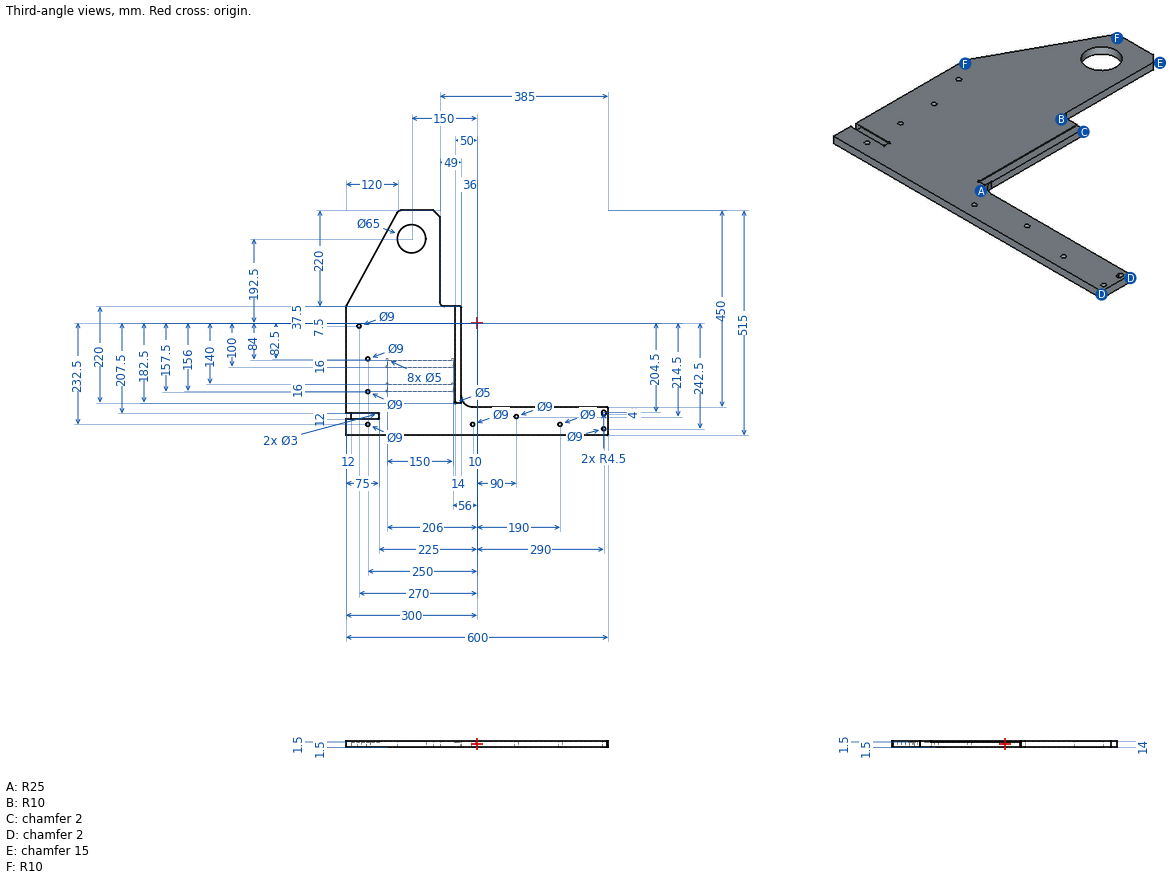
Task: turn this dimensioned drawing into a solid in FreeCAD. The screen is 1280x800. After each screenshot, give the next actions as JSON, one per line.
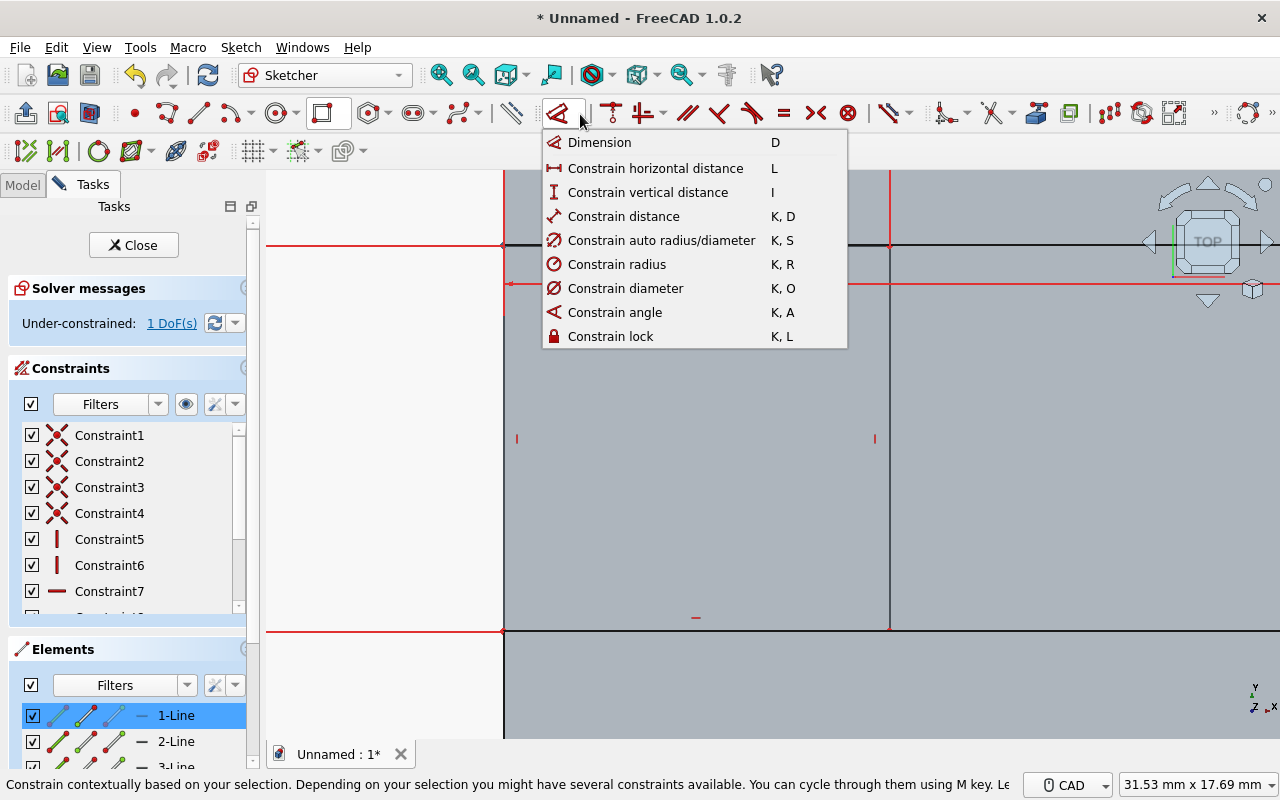
{"action": "left_click", "coordinate": [695, 192]}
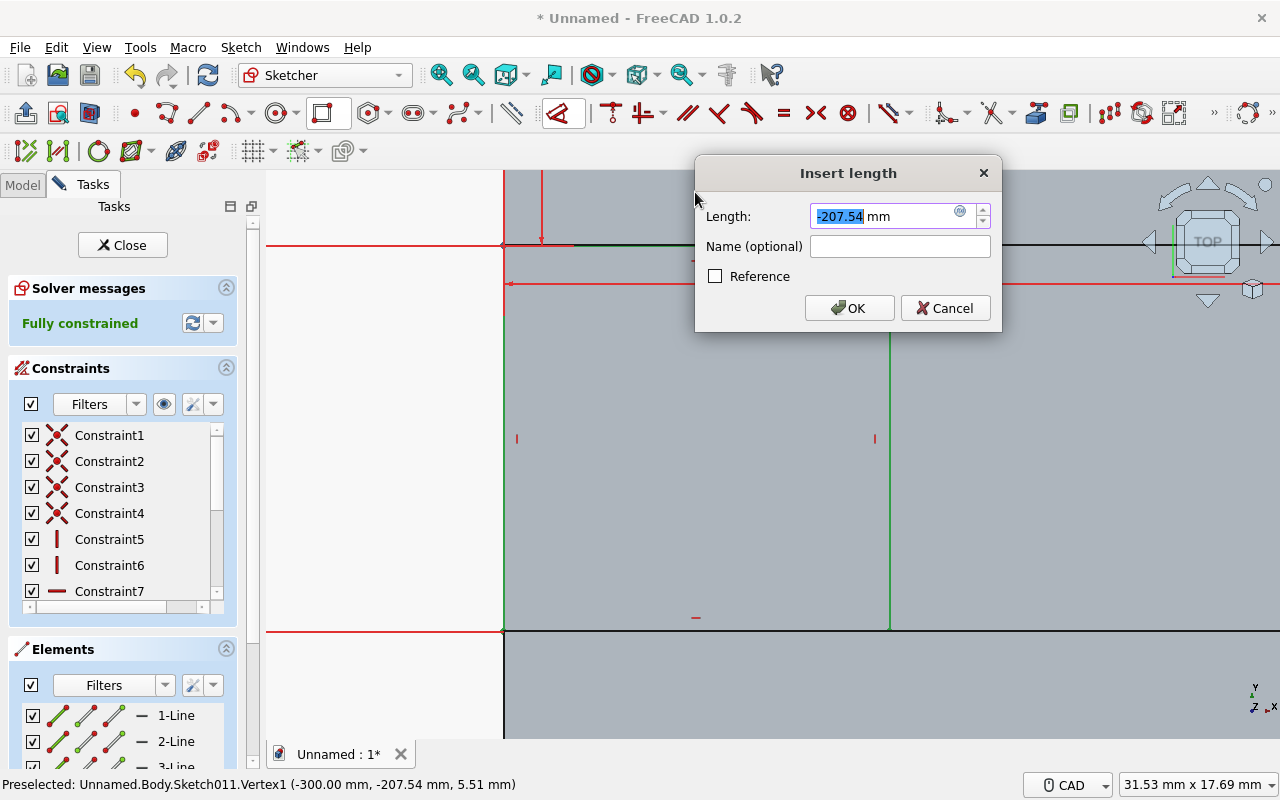
{"action": "type", "text": "-207.5"}
{"action": "key", "text": "Return"}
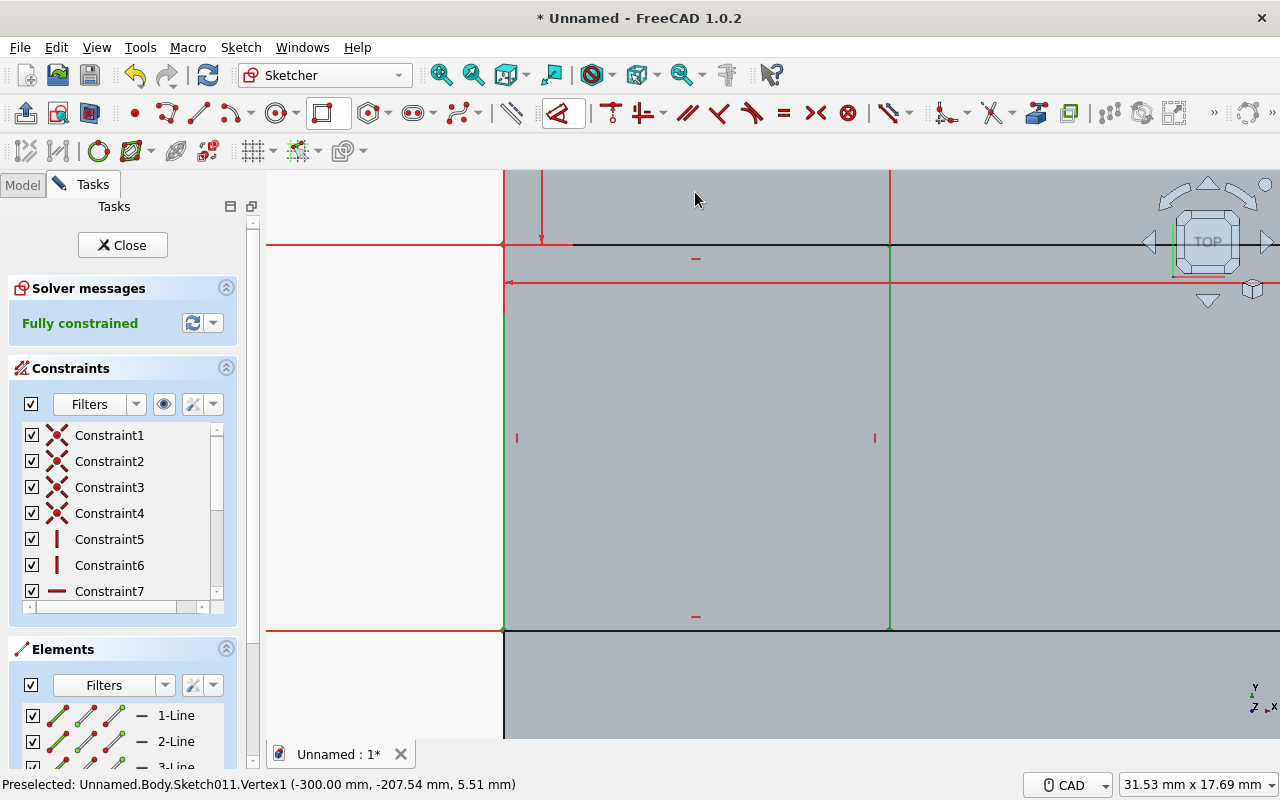
{"action": "left_click", "coordinate": [123, 245]}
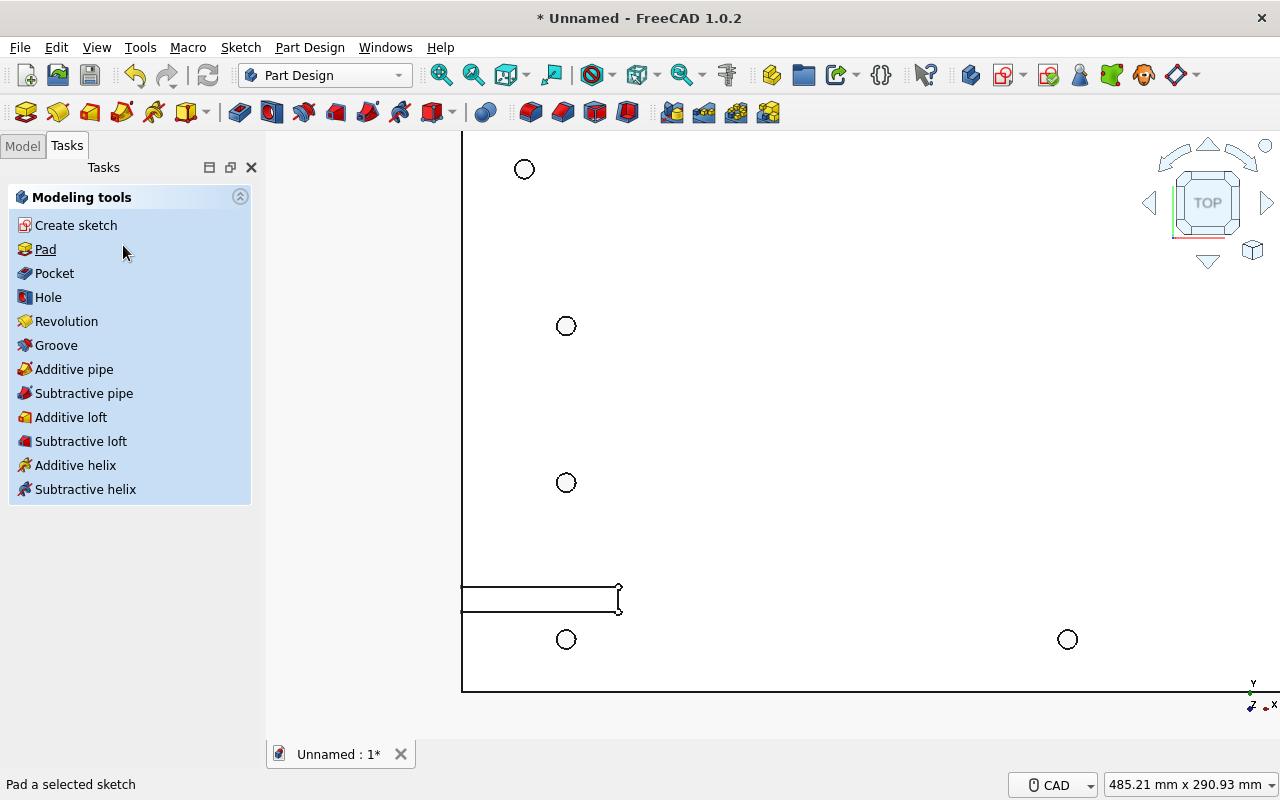
{"action": "left_click", "coordinate": [240, 112]}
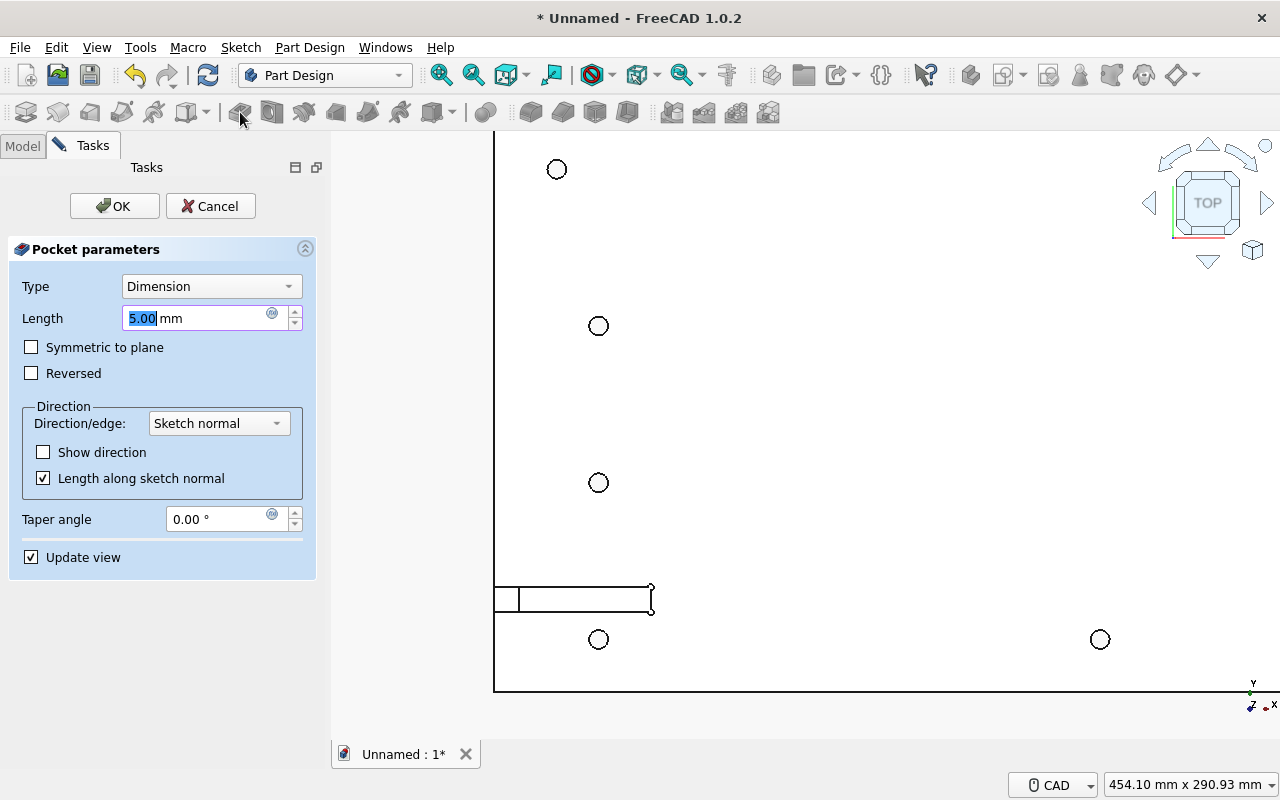
{"action": "left_click", "coordinate": [212, 286]}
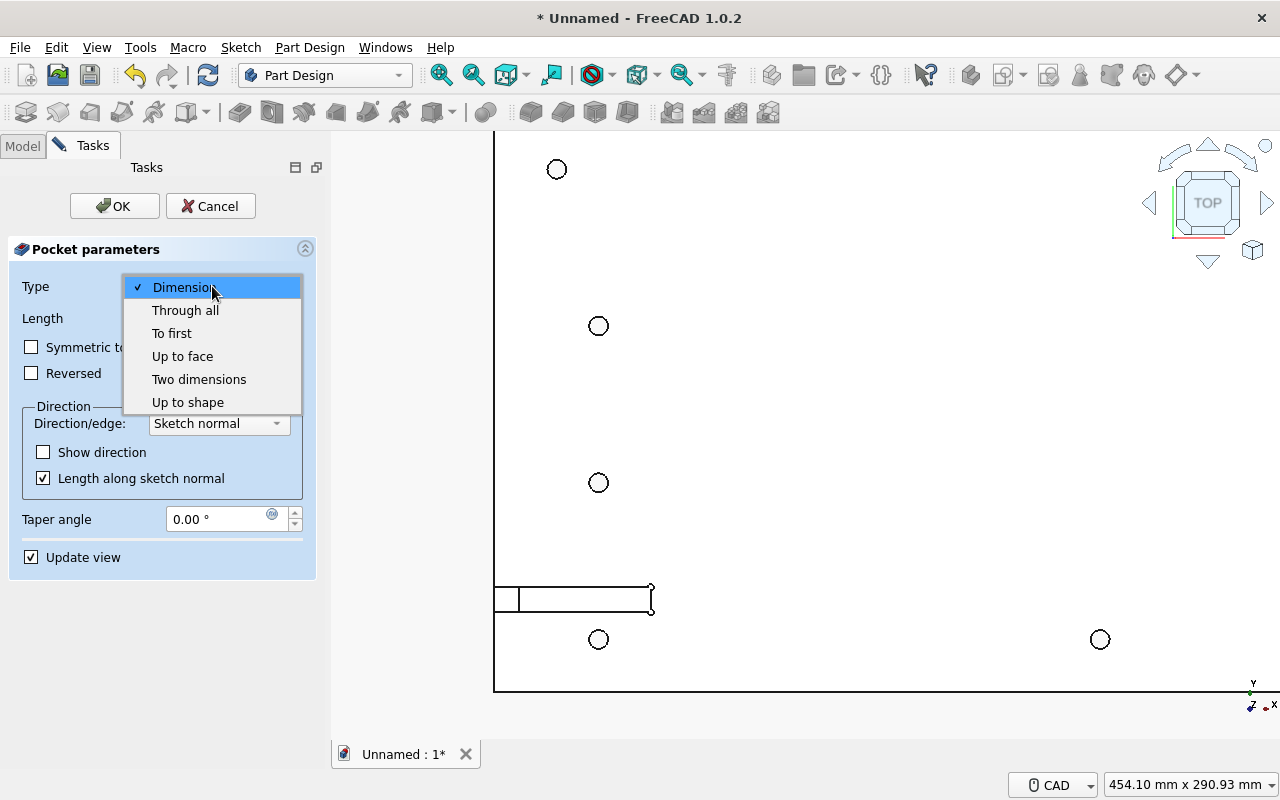
{"action": "left_click", "coordinate": [212, 334]}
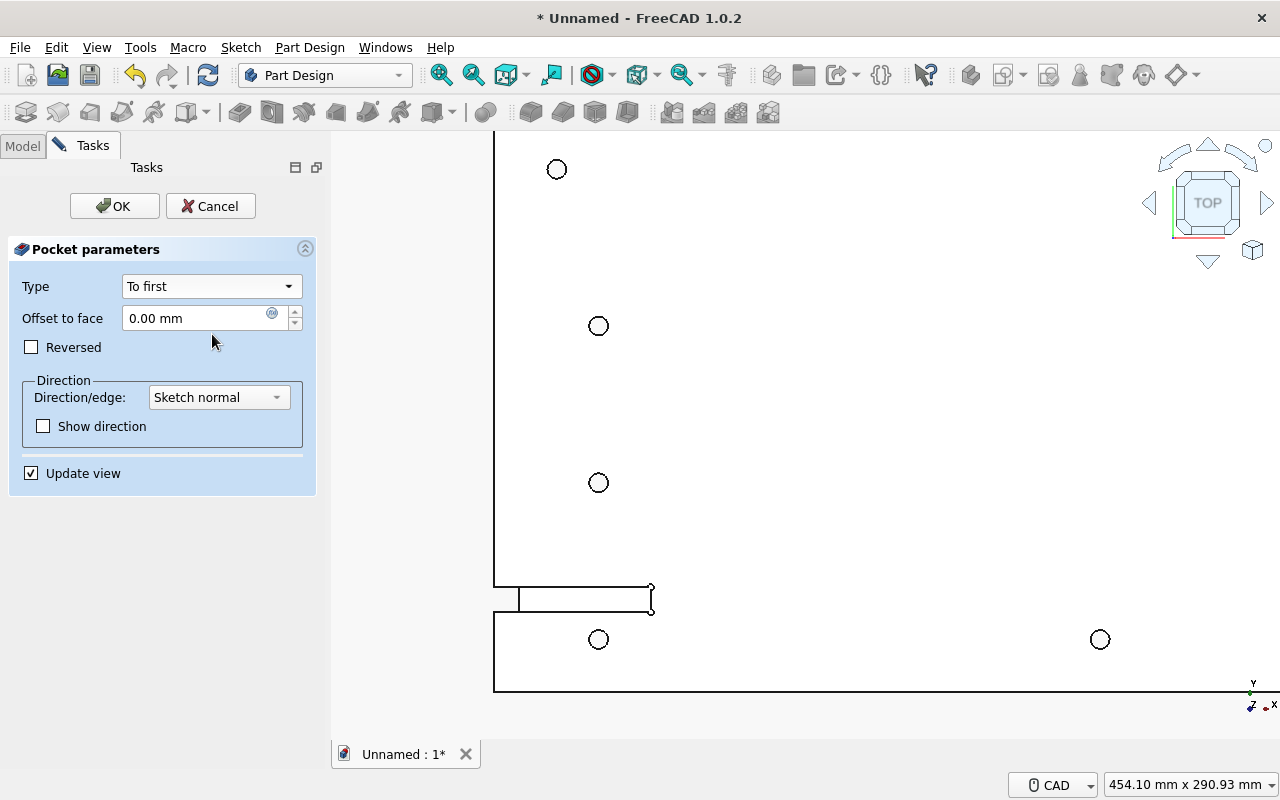
{"action": "left_click", "coordinate": [115, 206]}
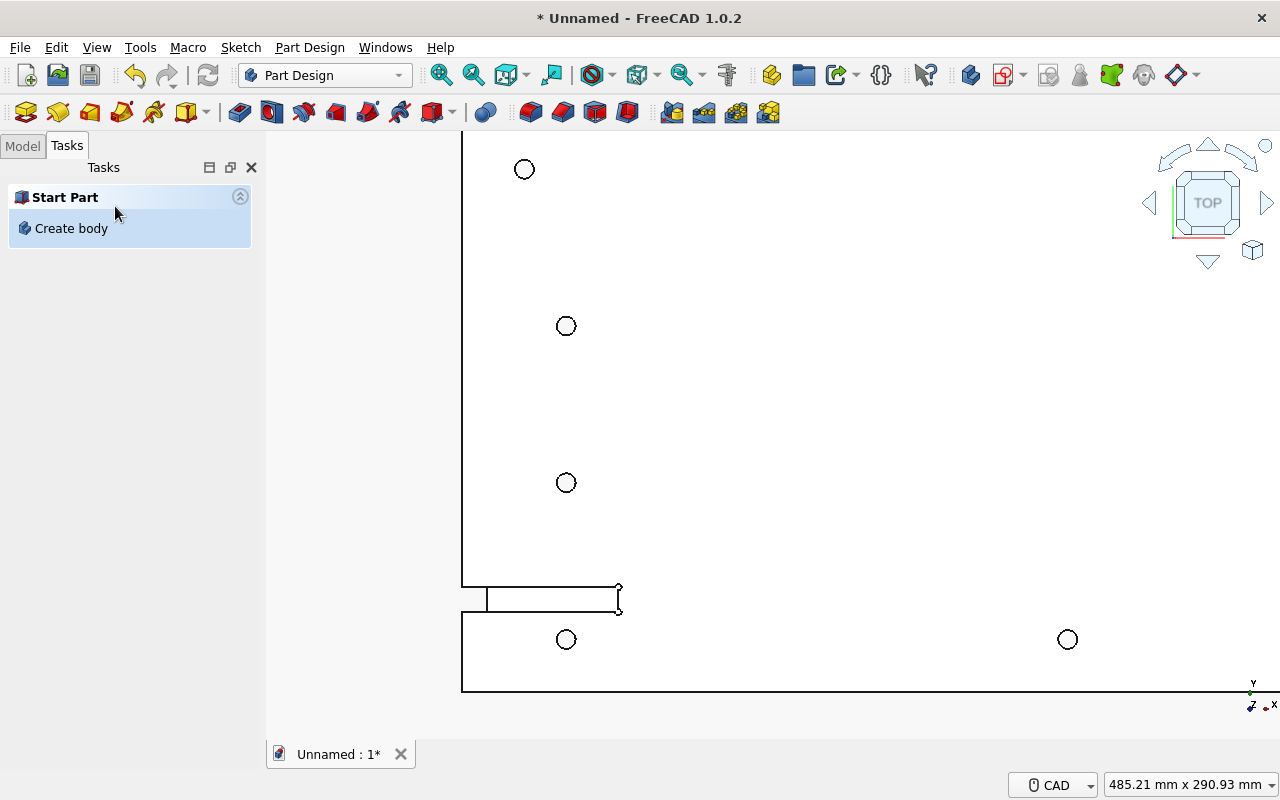
{"action": "left_click", "coordinate": [442, 76]}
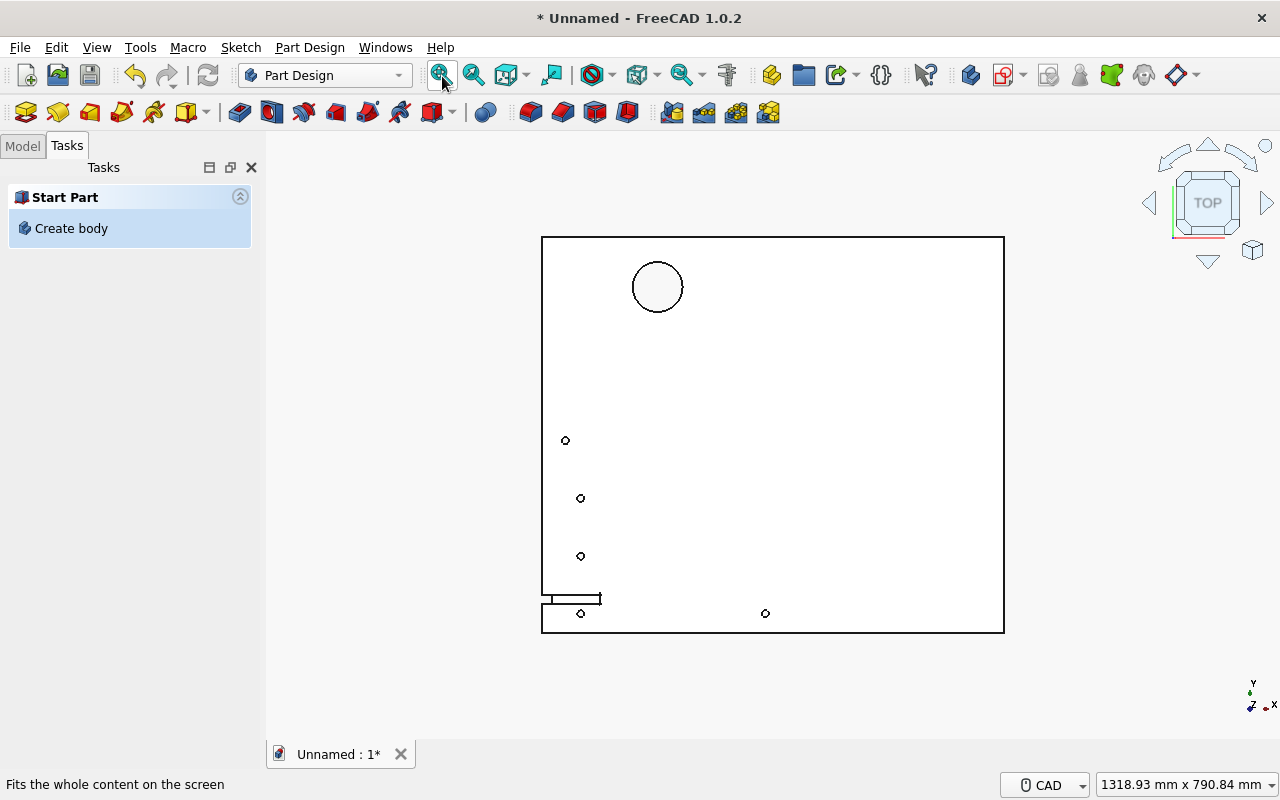
{"action": "key", "text": "5"}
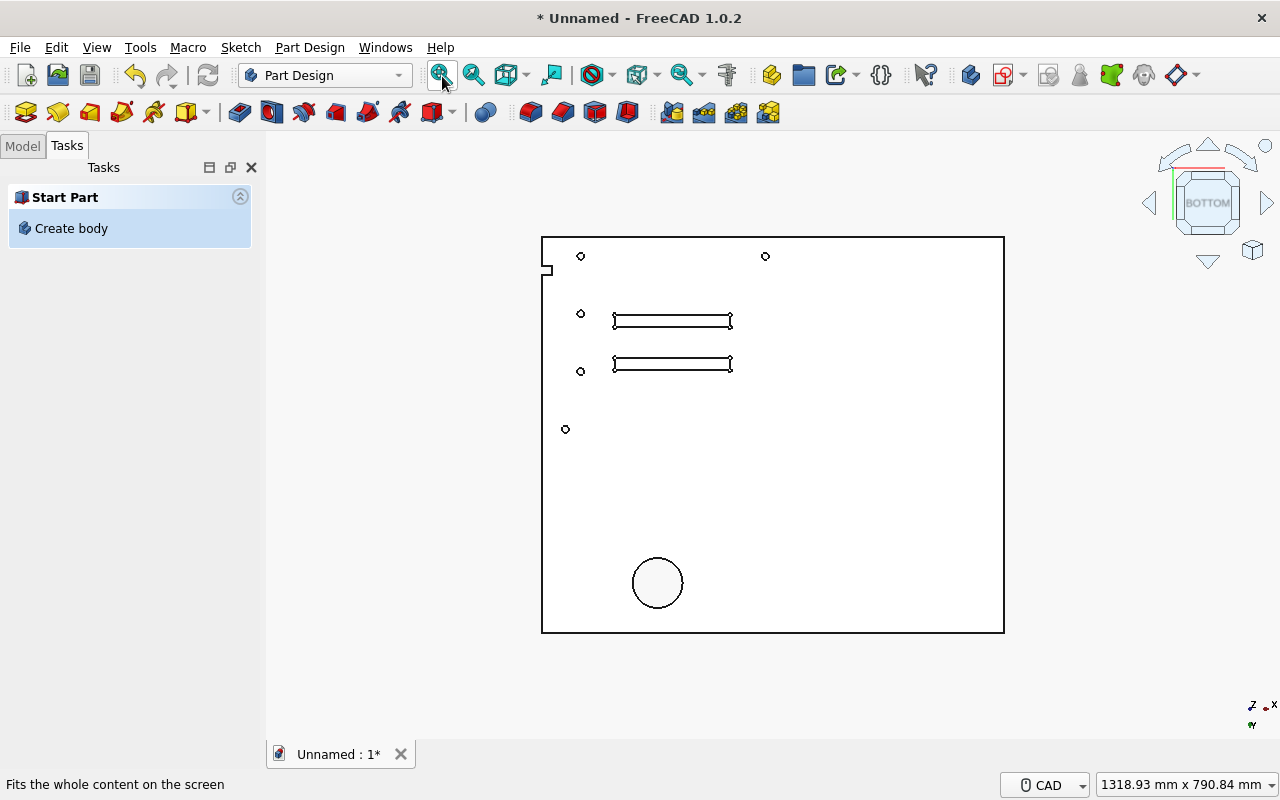
{"action": "left_click", "coordinate": [839, 491]}